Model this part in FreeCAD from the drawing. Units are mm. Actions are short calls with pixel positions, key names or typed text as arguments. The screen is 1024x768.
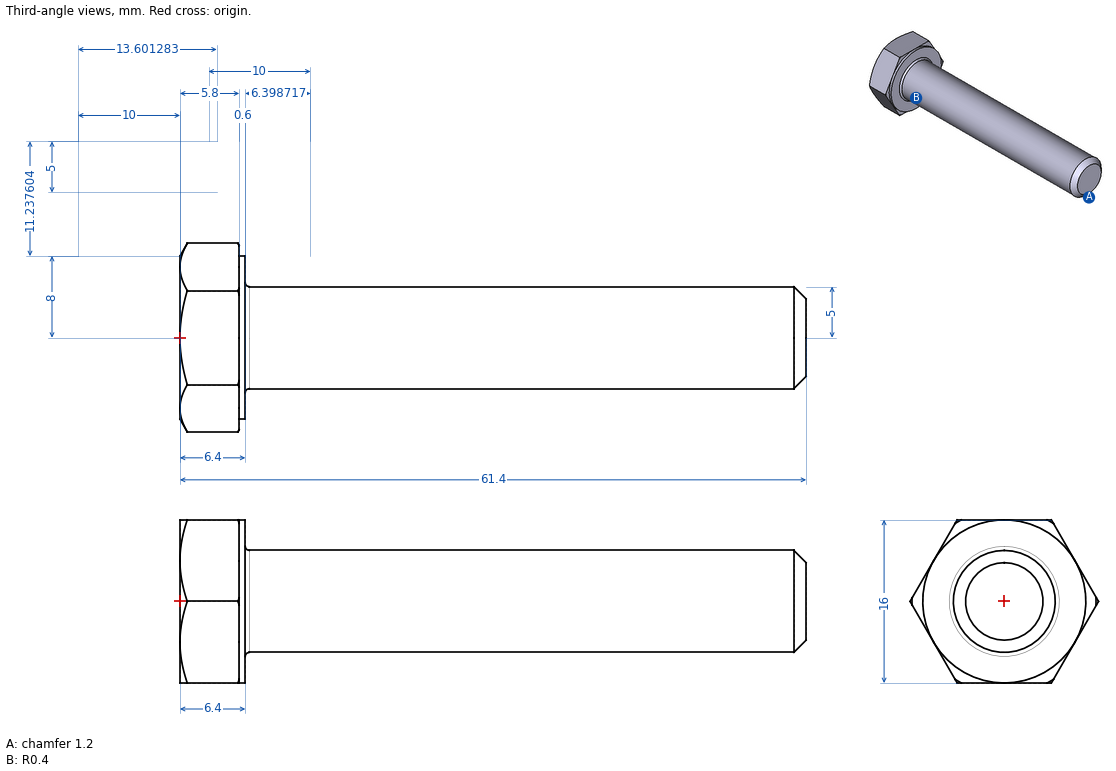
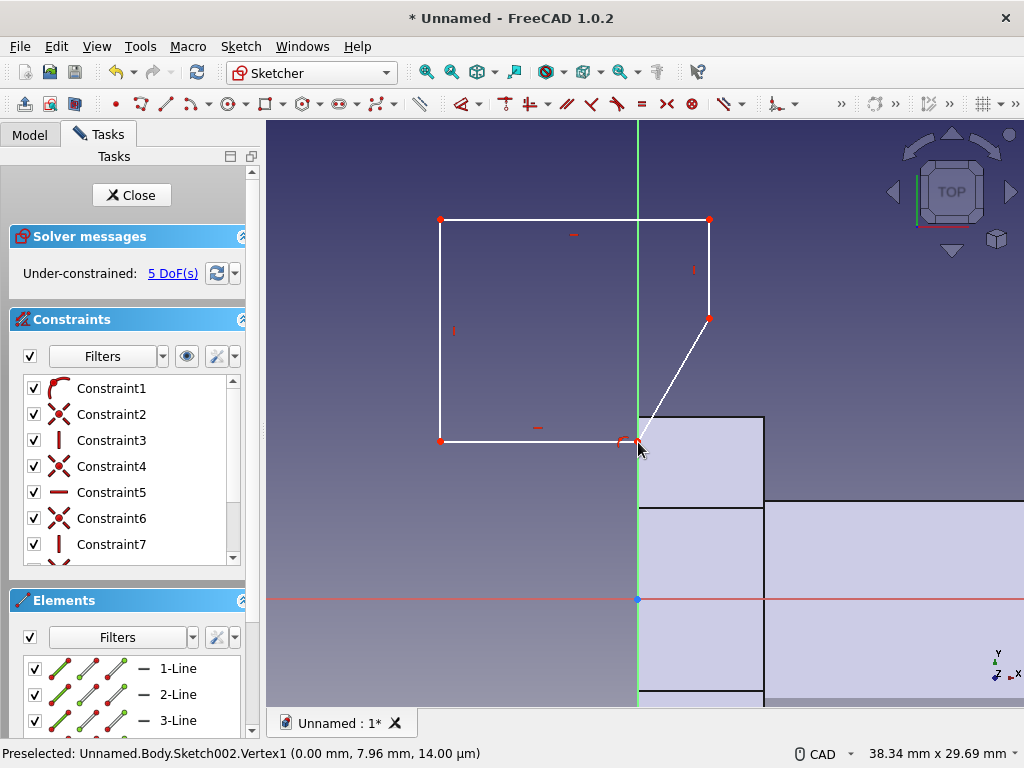
click(709, 289)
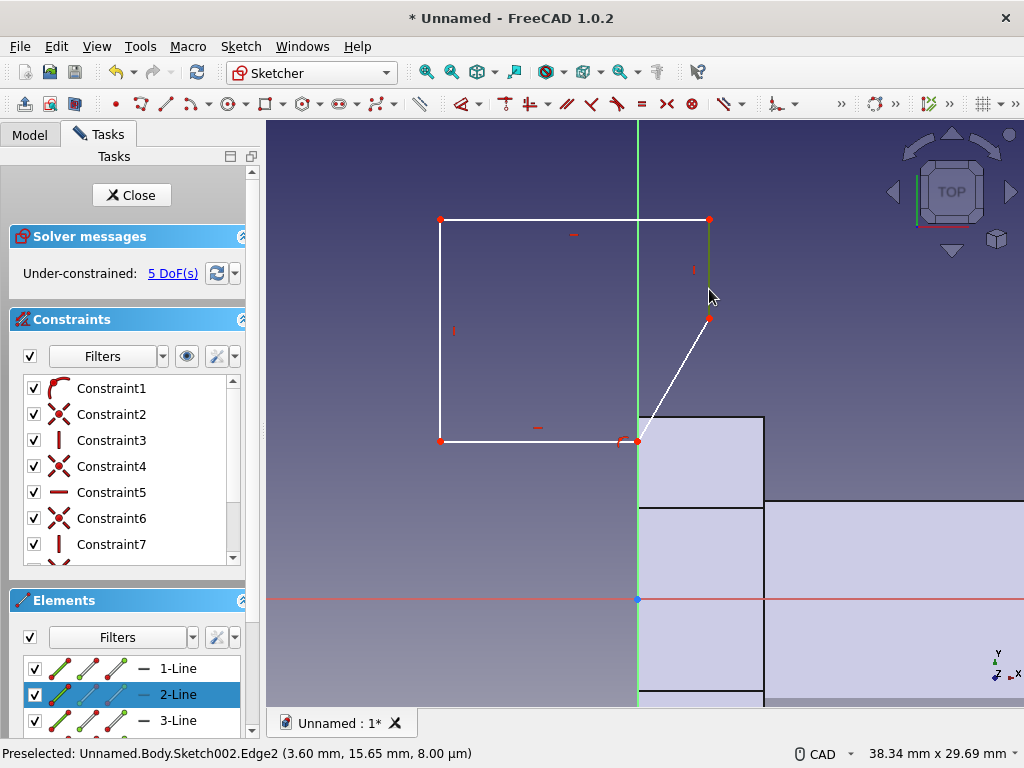
key(i)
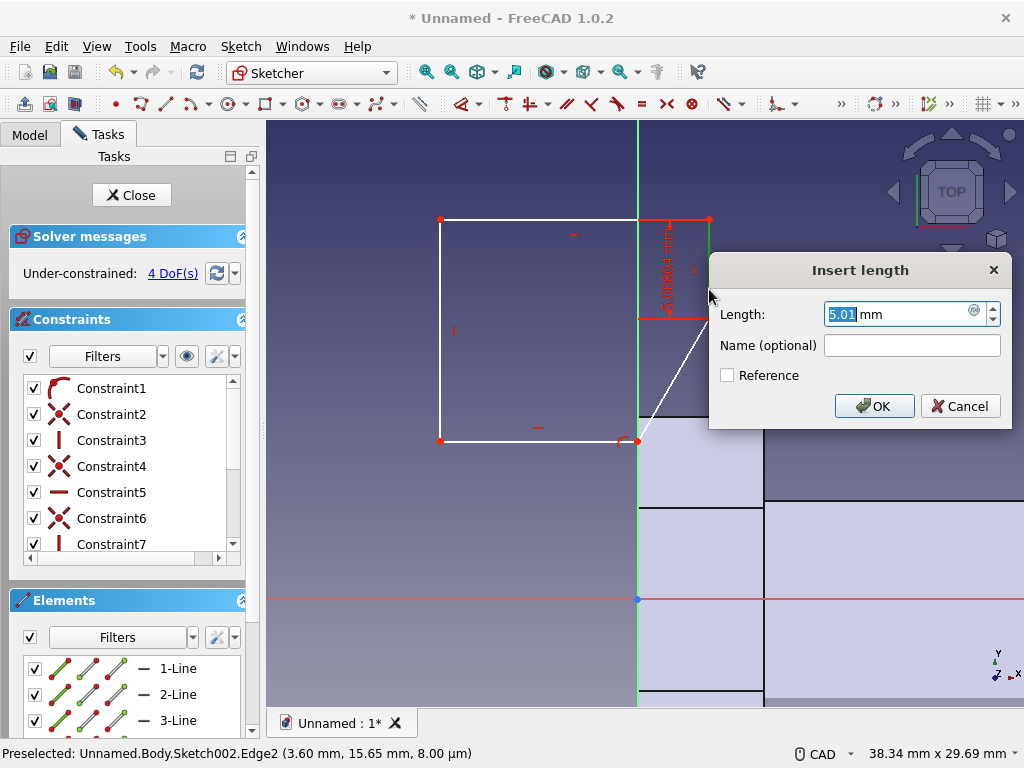
text(5)
key(Return)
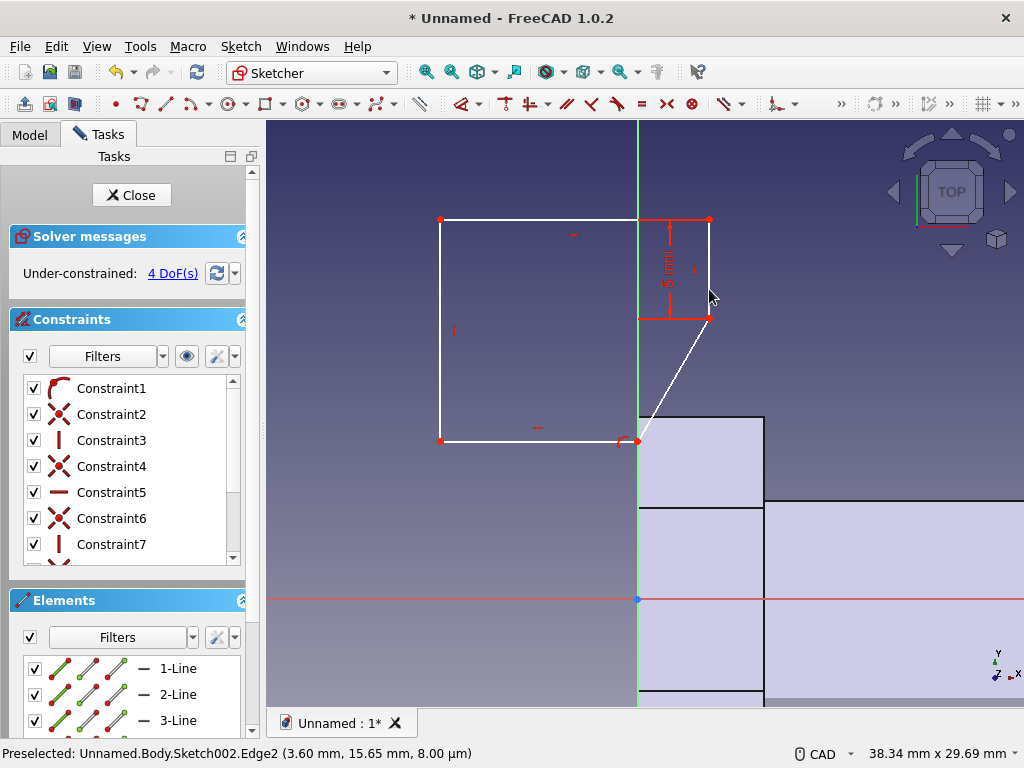
click(499, 442)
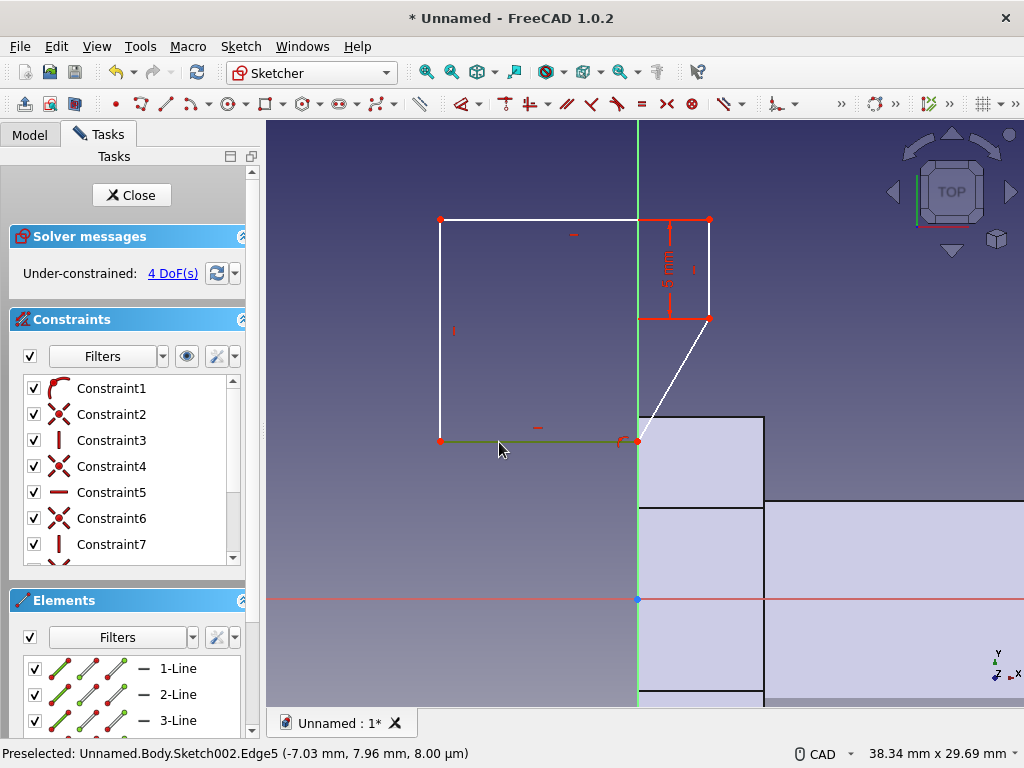
click(478, 104)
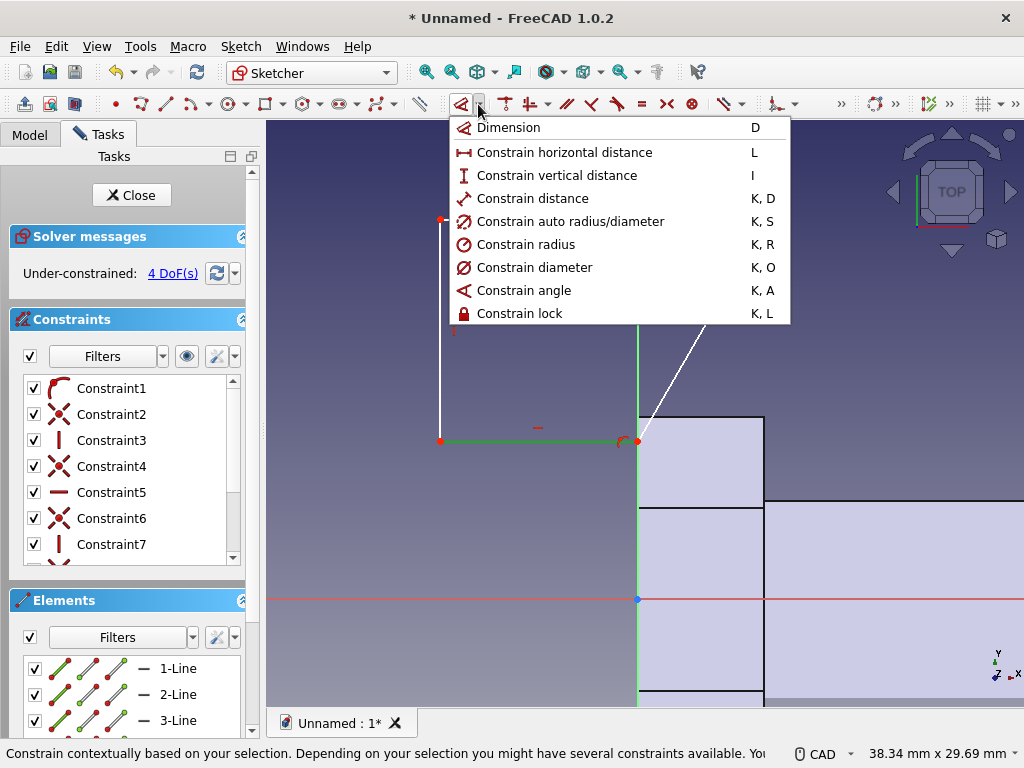
click(620, 152)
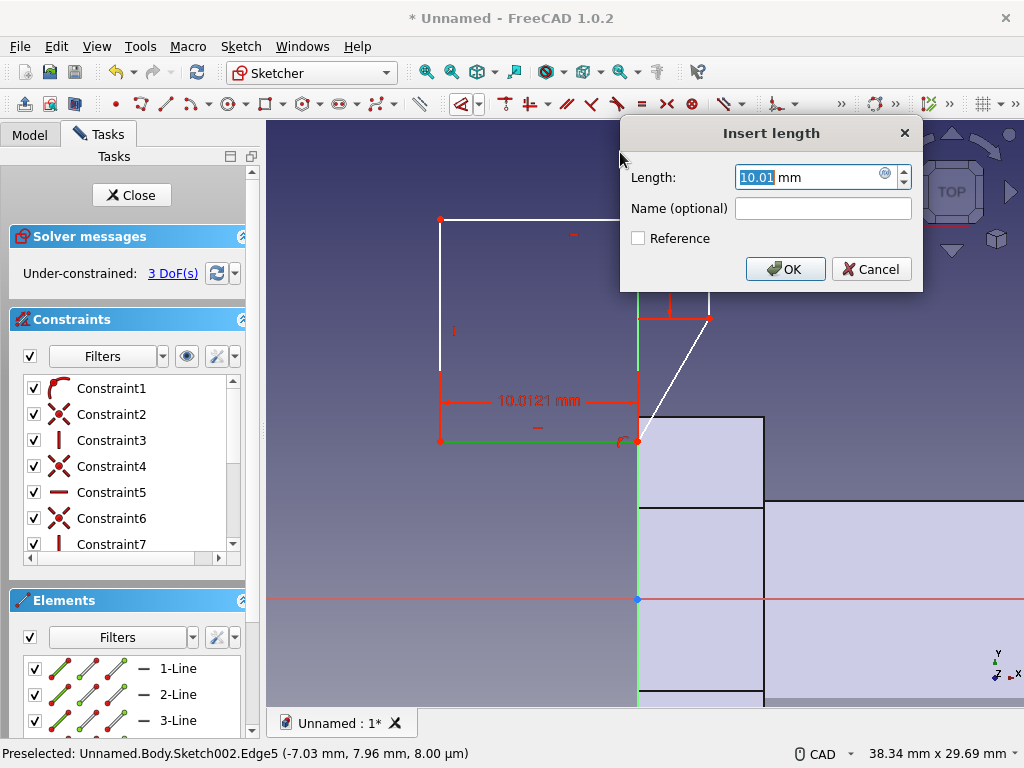
text(10)
key(Return)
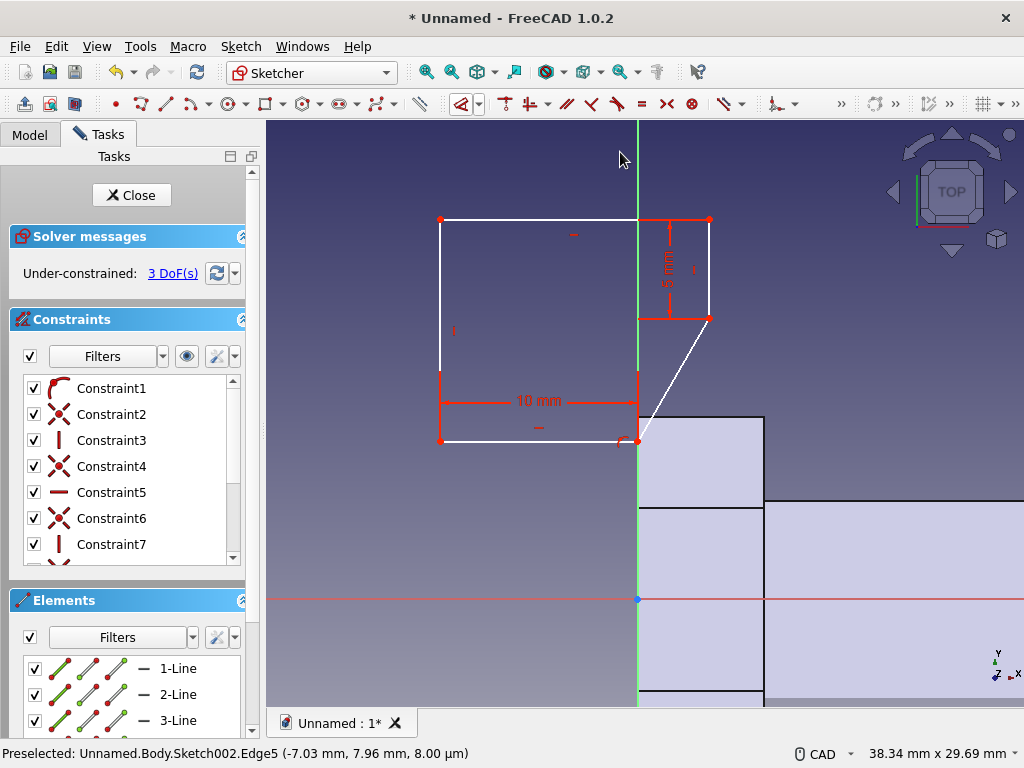
click(638, 442)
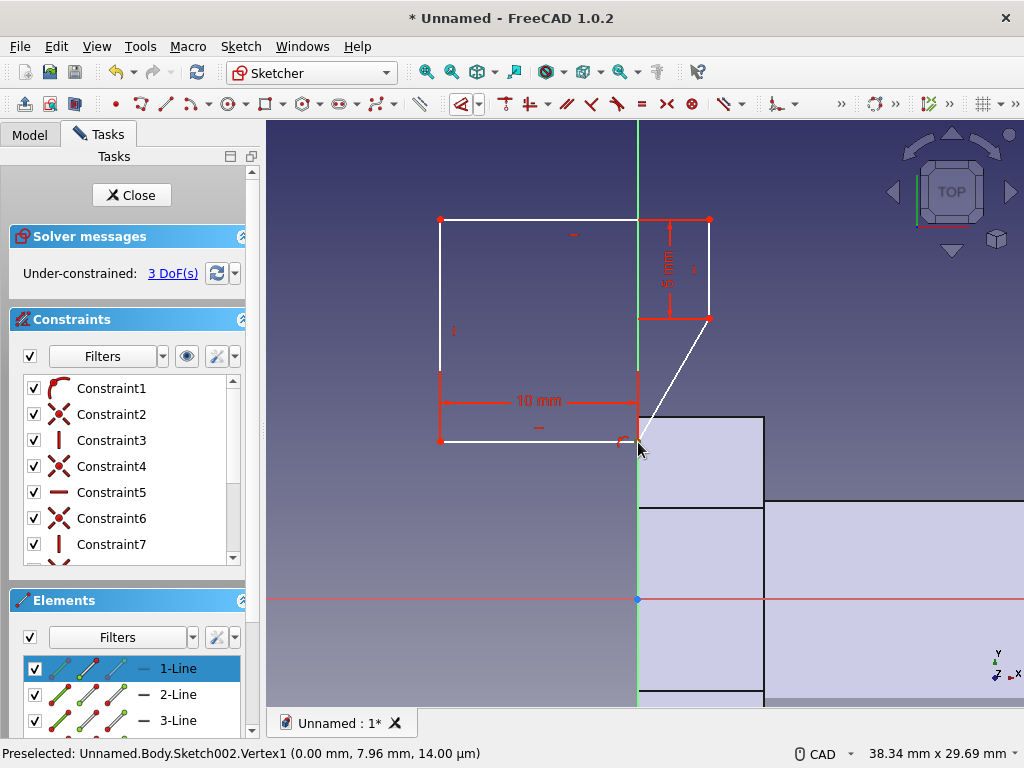
key(i)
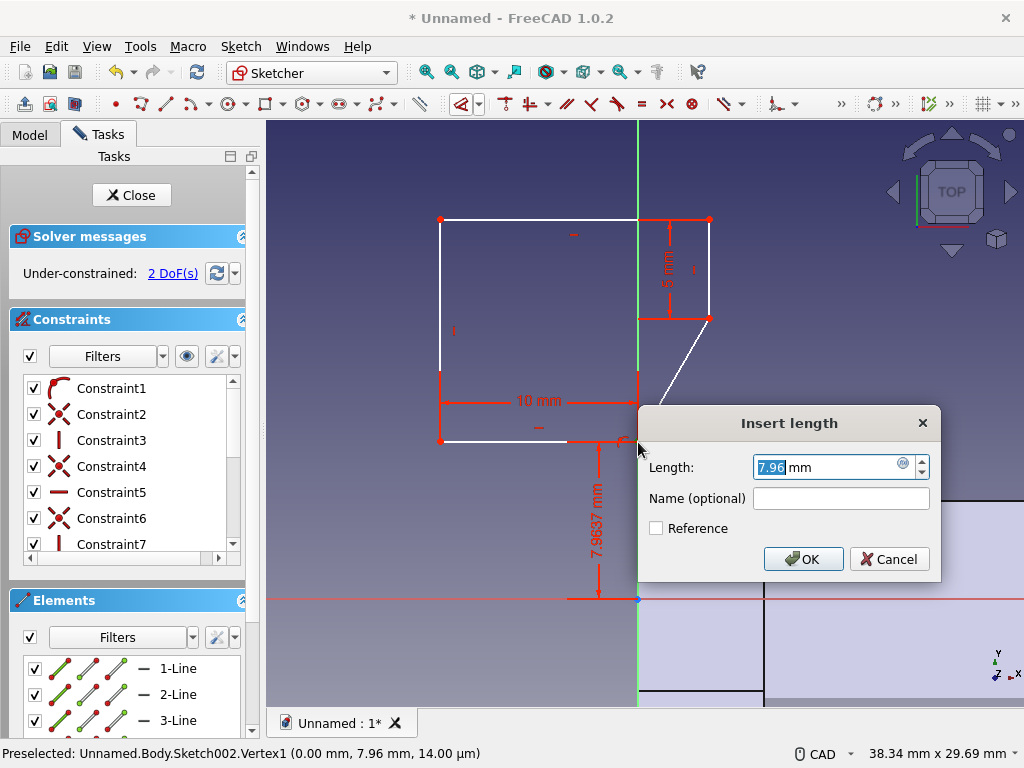
text(8)
key(Return)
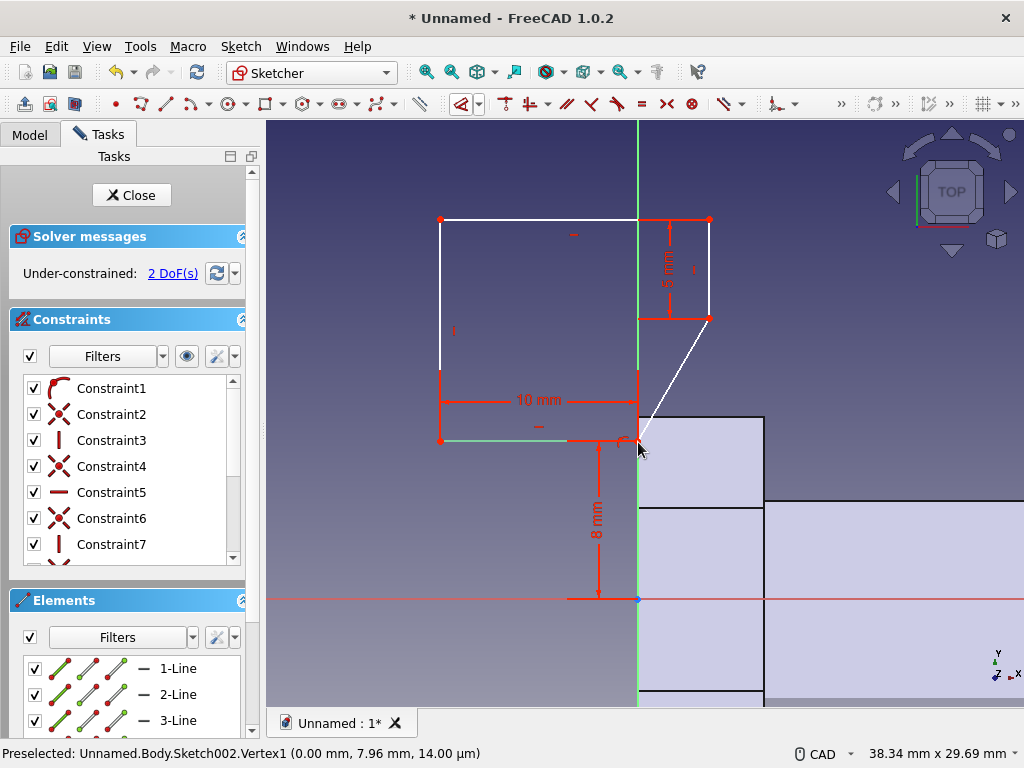
scroll(628, 220, up, 2)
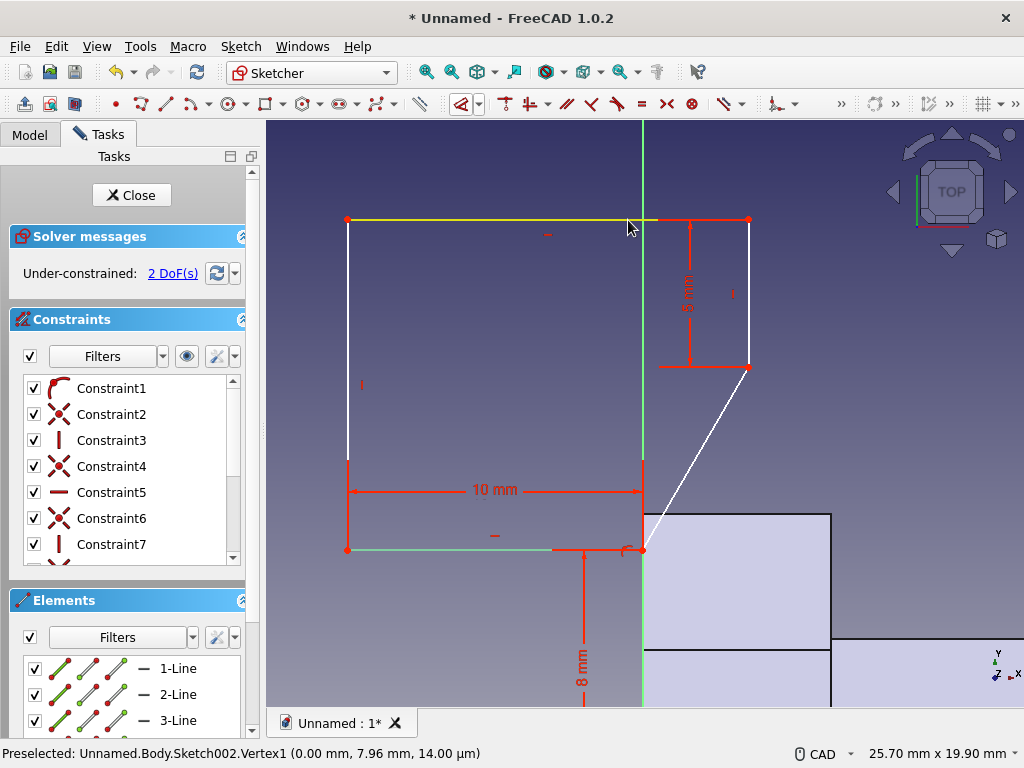
click(628, 220)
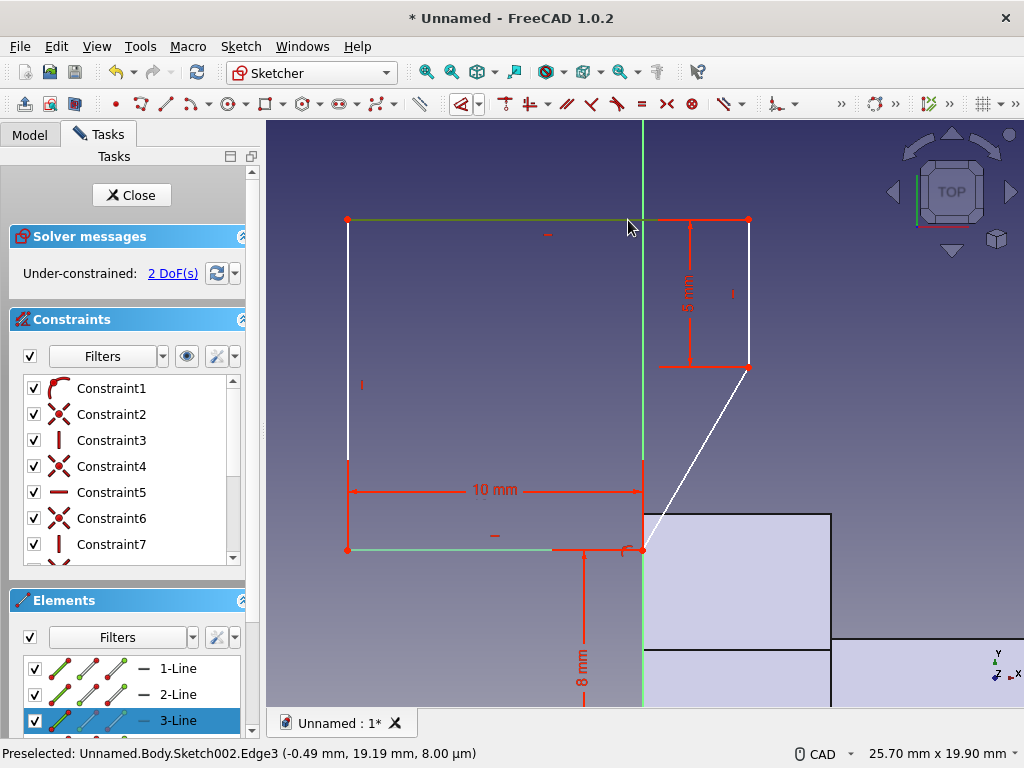
key(l)